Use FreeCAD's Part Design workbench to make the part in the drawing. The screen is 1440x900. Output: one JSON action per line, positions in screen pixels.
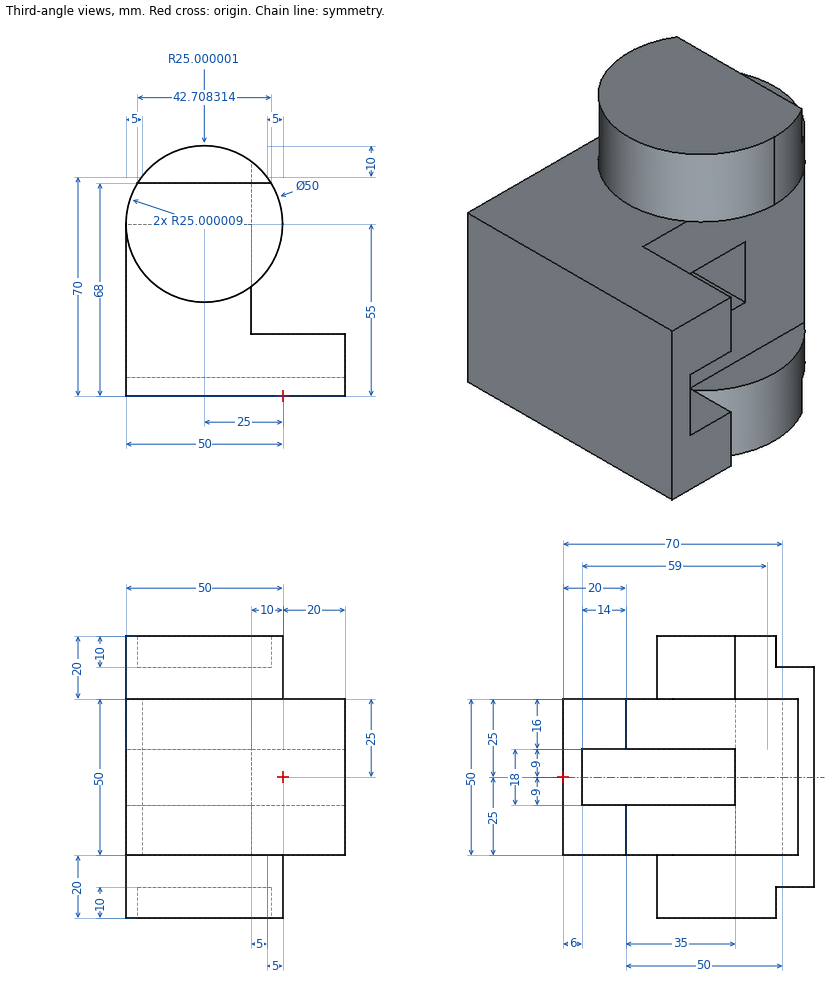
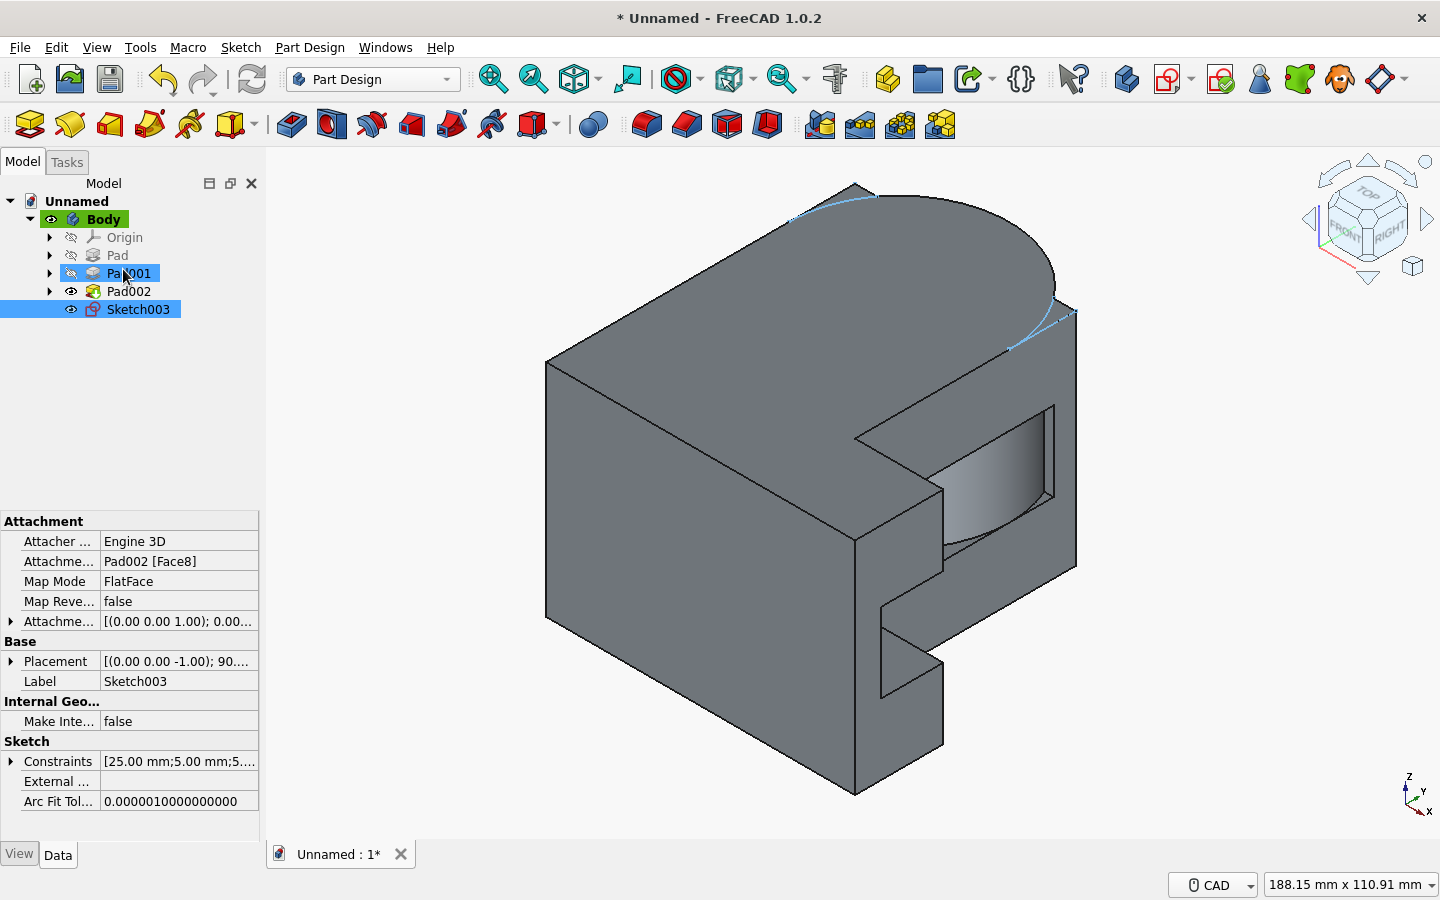
{"action": "left_click", "coordinate": [292, 124]}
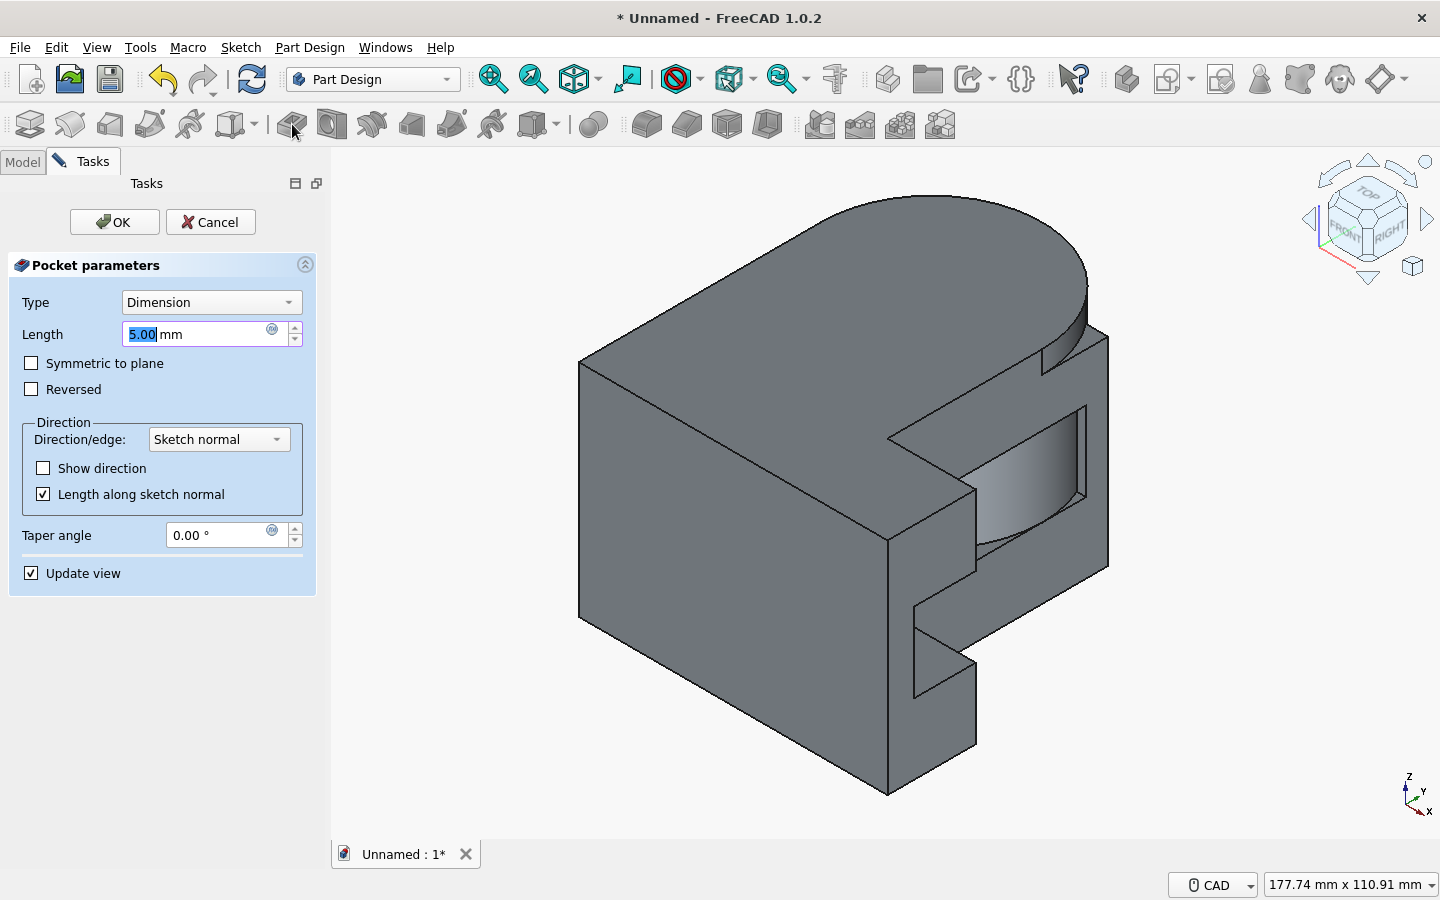
{"action": "type", "text": "50"}
{"action": "key", "text": "Tab"}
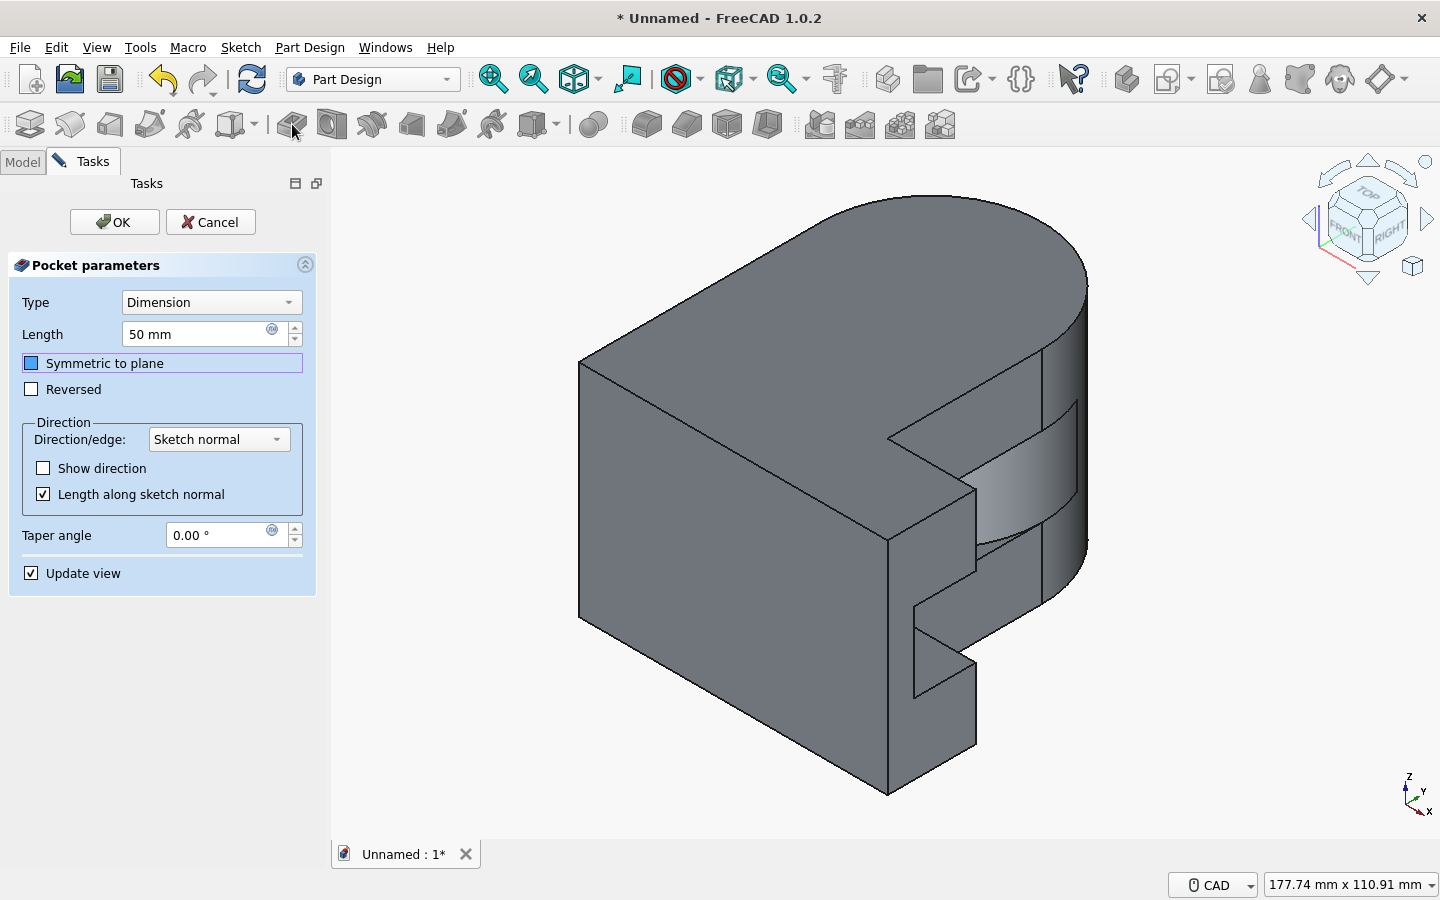
{"action": "left_click", "coordinate": [115, 222]}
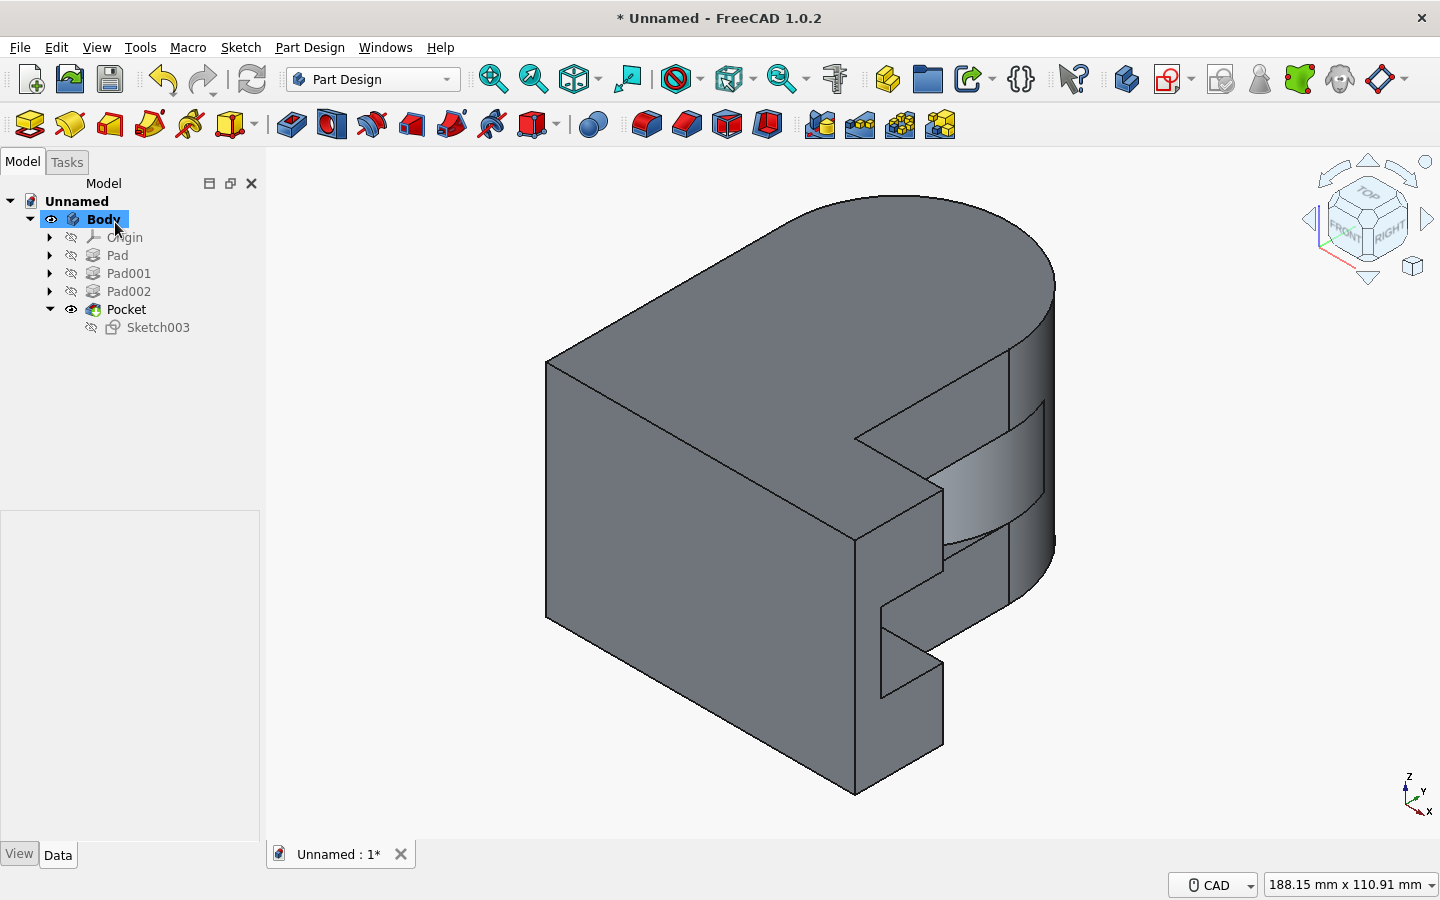
{"action": "left_click", "coordinate": [932, 607]}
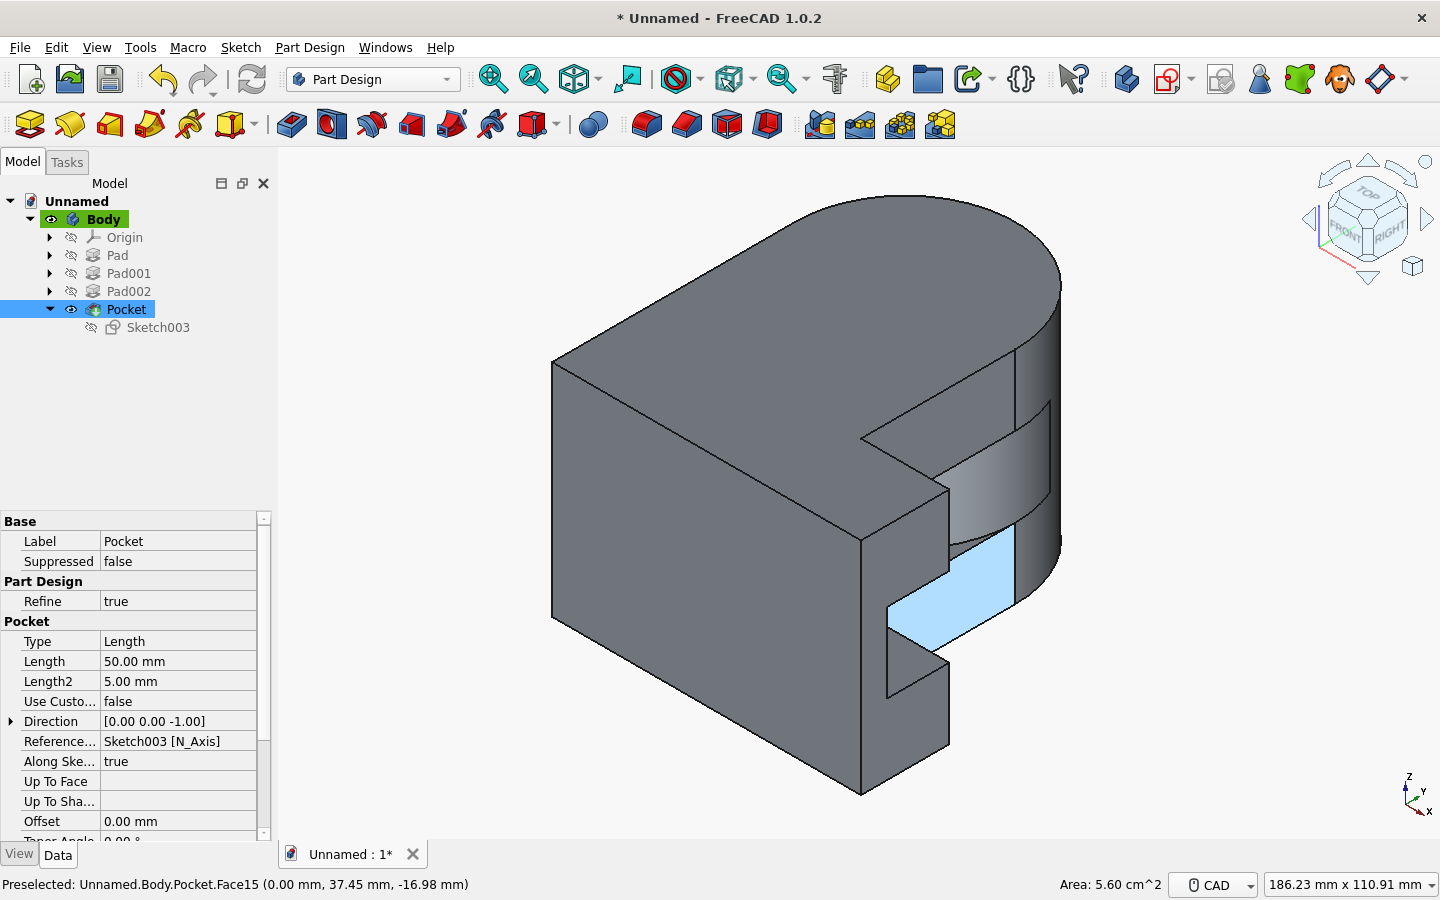
{"action": "left_click", "coordinate": [1168, 80]}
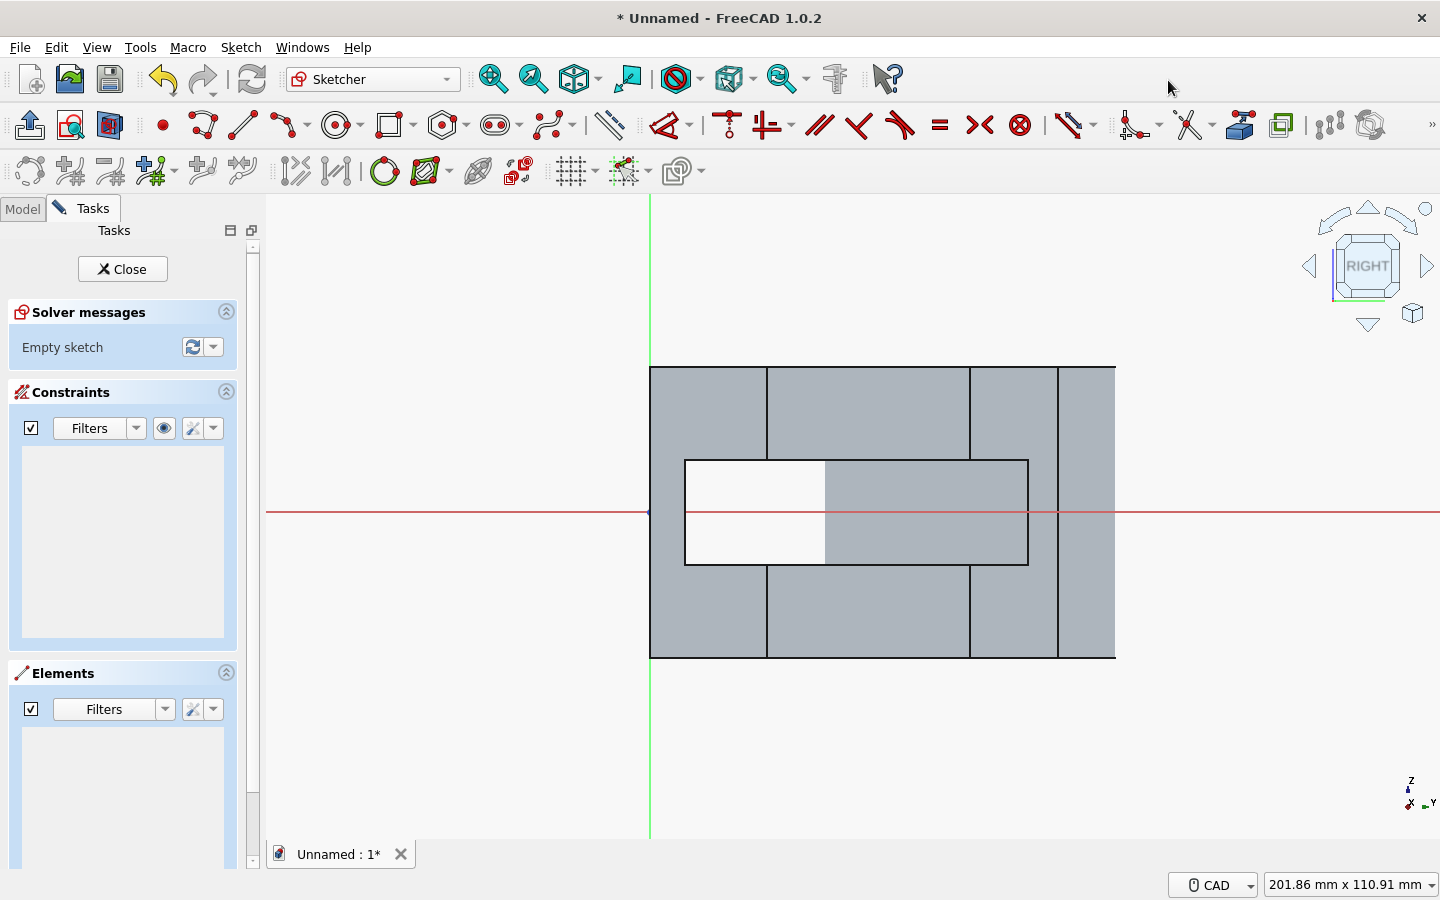
{"action": "scroll", "coordinate": [832, 509], "scroll_direction": "up", "scroll_amount": 4}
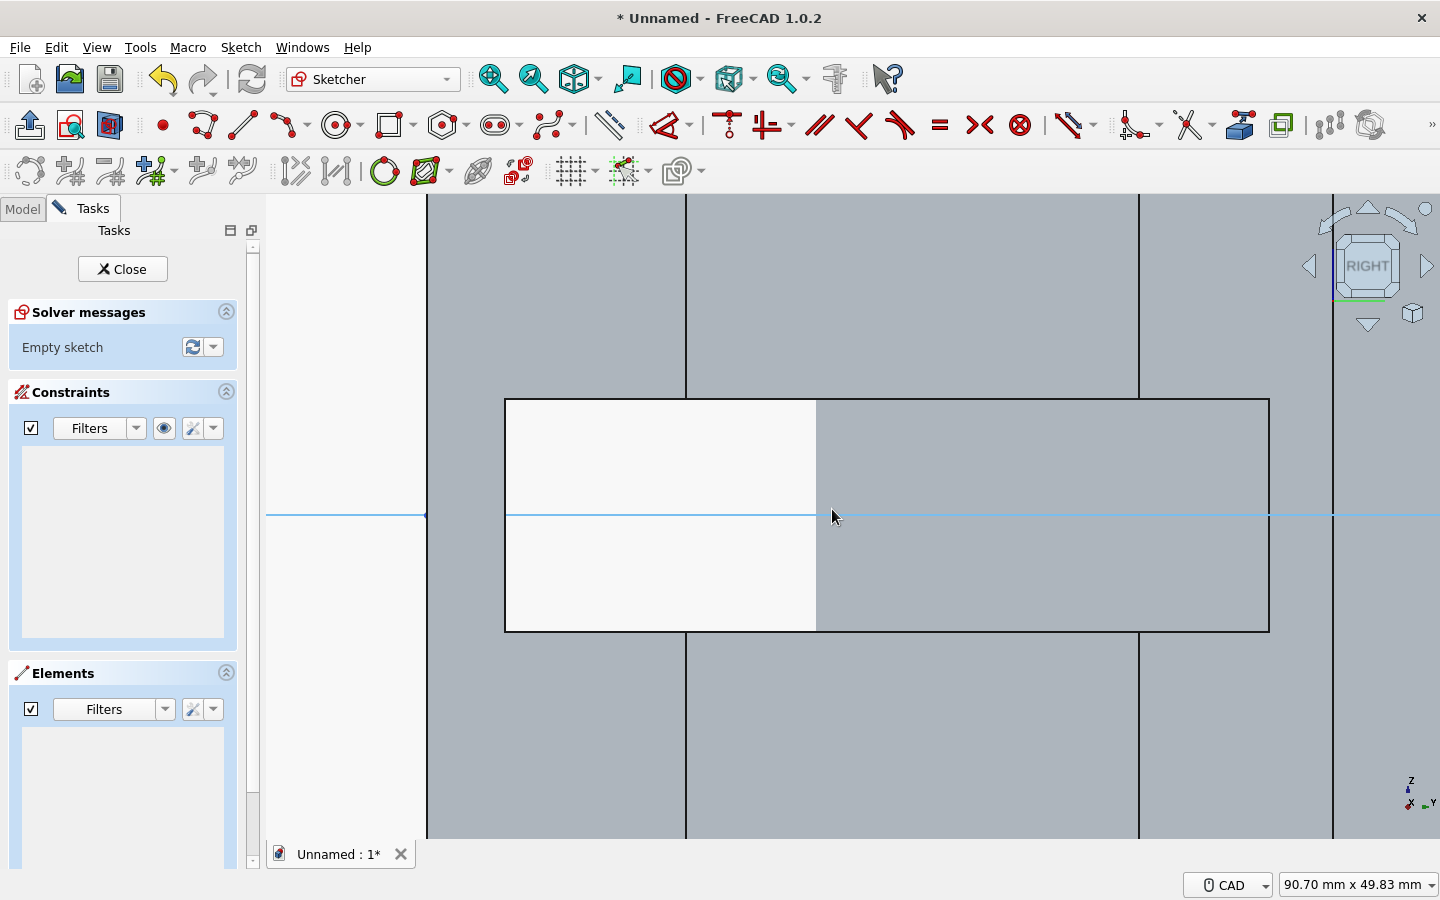
{"action": "left_click", "coordinate": [390, 126]}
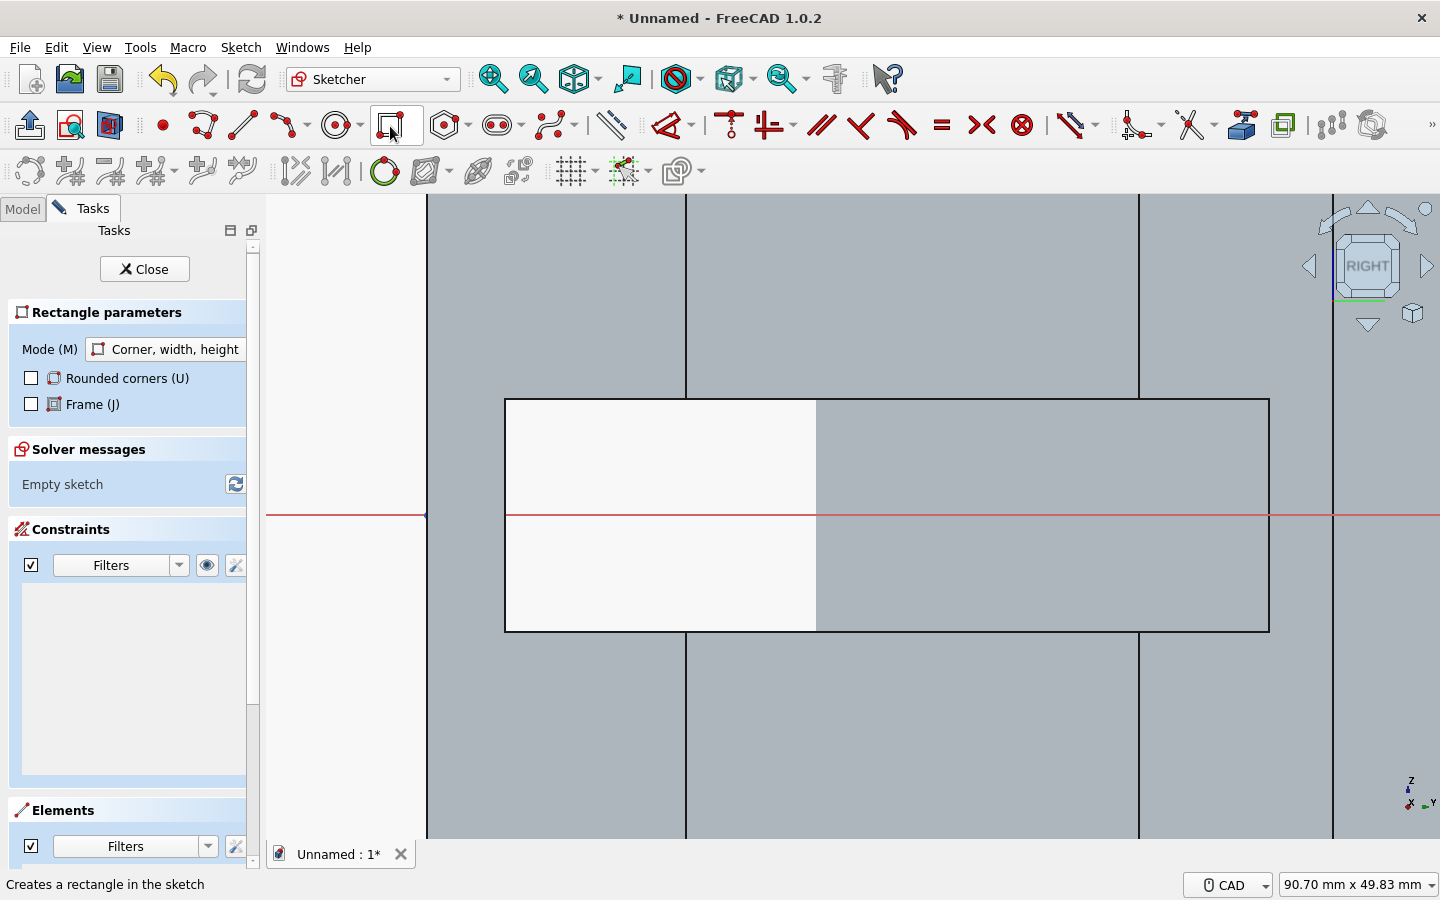
{"action": "left_click", "coordinate": [686, 399]}
{"action": "mouse_move", "coordinate": [1139, 632]}